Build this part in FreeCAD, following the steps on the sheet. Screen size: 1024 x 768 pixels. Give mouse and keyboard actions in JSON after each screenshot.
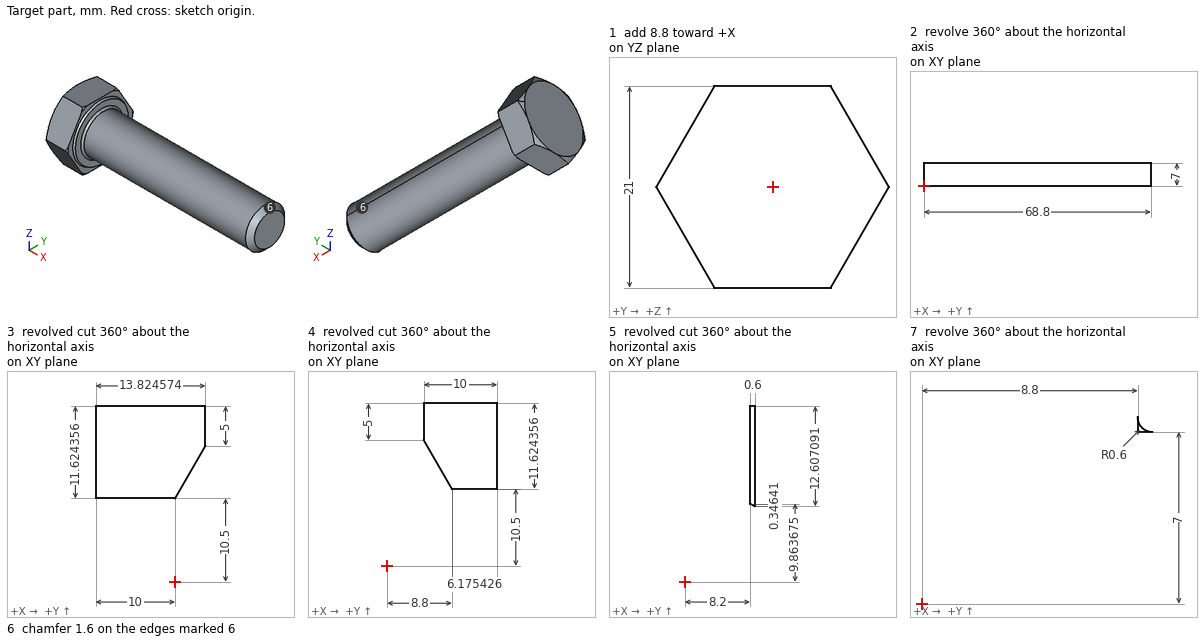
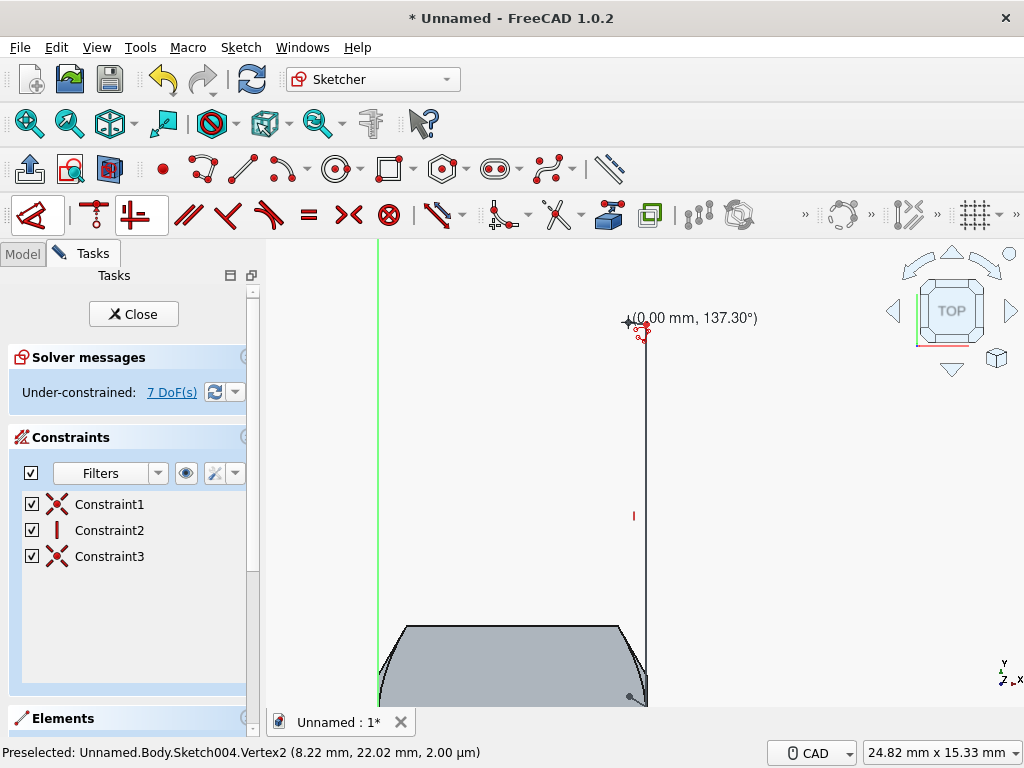
{"action": "scroll", "coordinate": [629, 322], "scroll_direction": "down", "scroll_amount": 4}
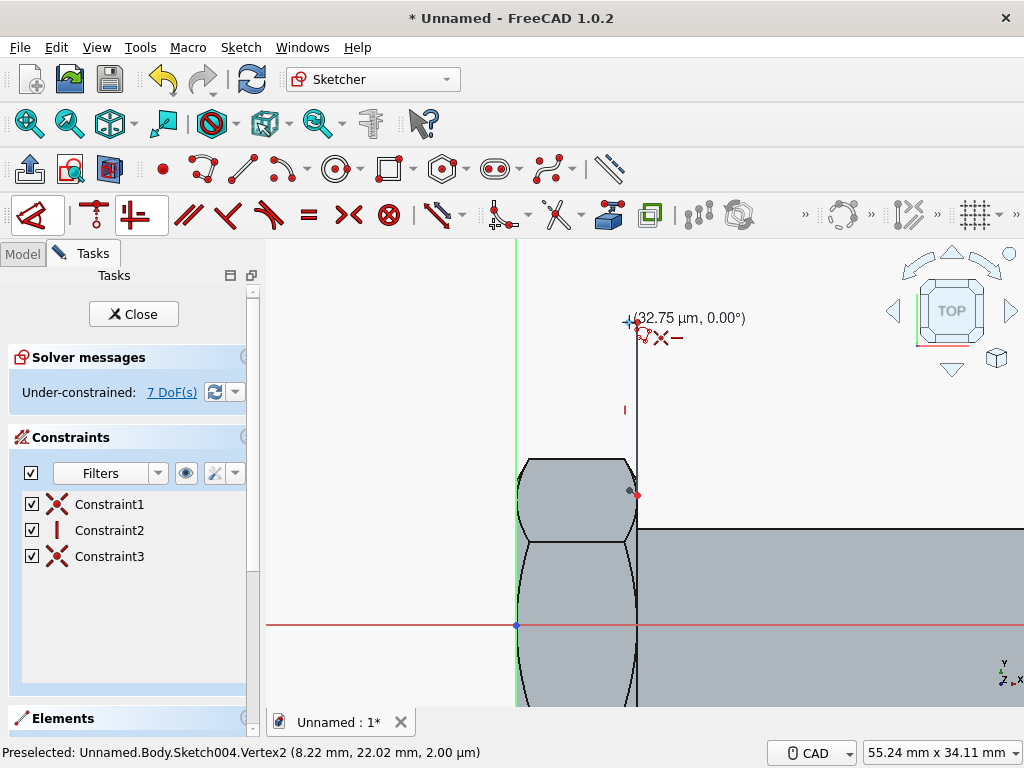
{"action": "scroll", "coordinate": [629, 490], "scroll_direction": "up", "scroll_amount": 7}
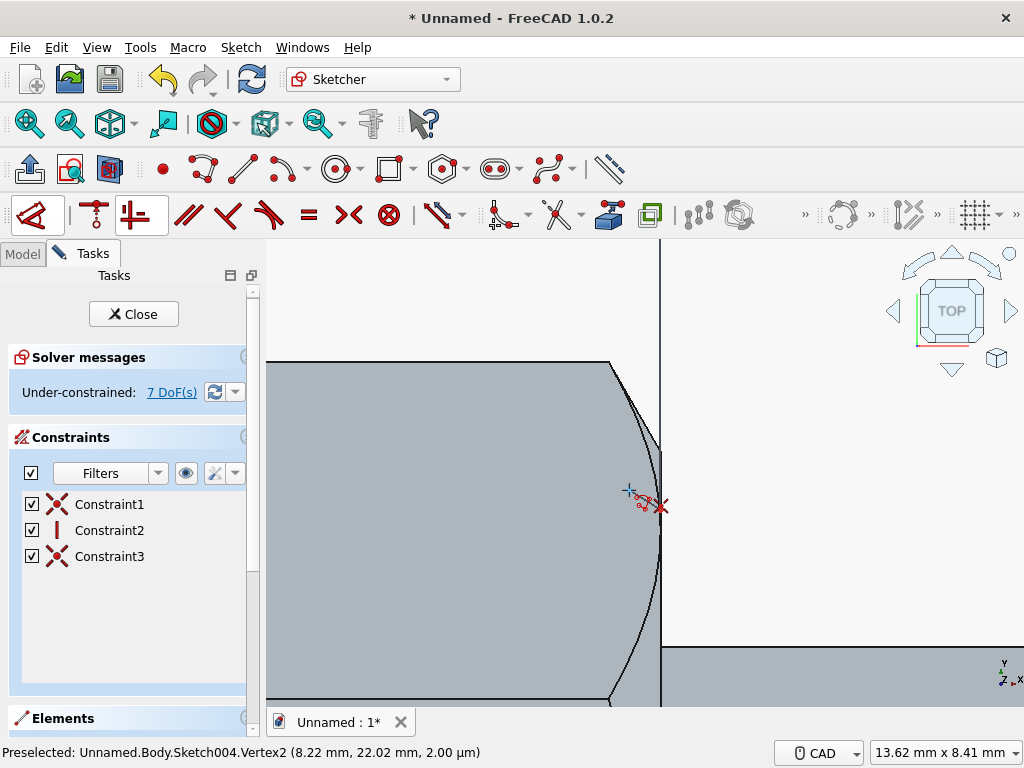
{"action": "left_click", "coordinate": [629, 490]}
{"action": "key", "text": "Escape"}
{"action": "key", "text": "Escape"}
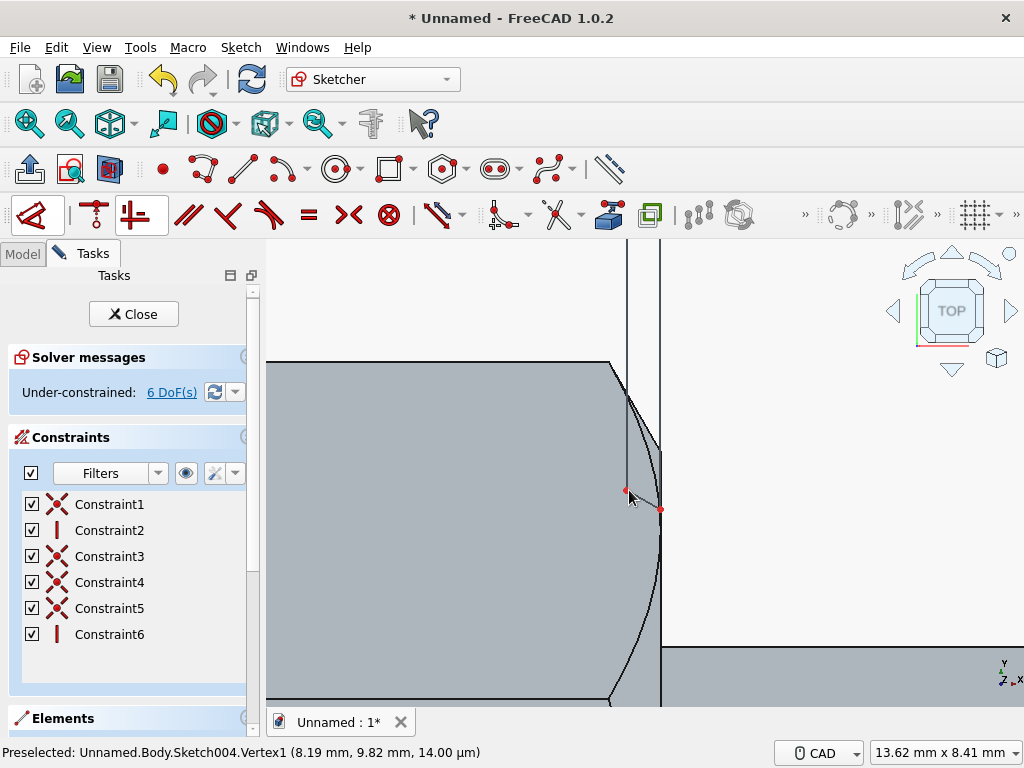
{"action": "scroll", "coordinate": [629, 490], "scroll_direction": "down", "scroll_amount": 7}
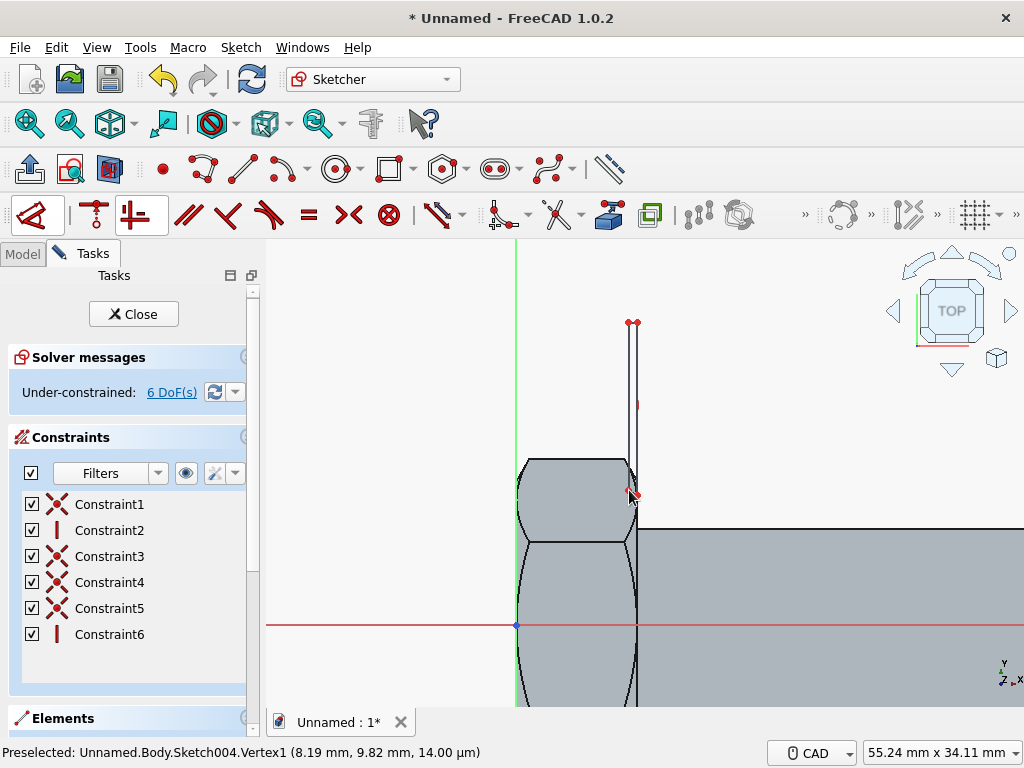
{"action": "scroll", "coordinate": [635, 323], "scroll_direction": "up", "scroll_amount": 9}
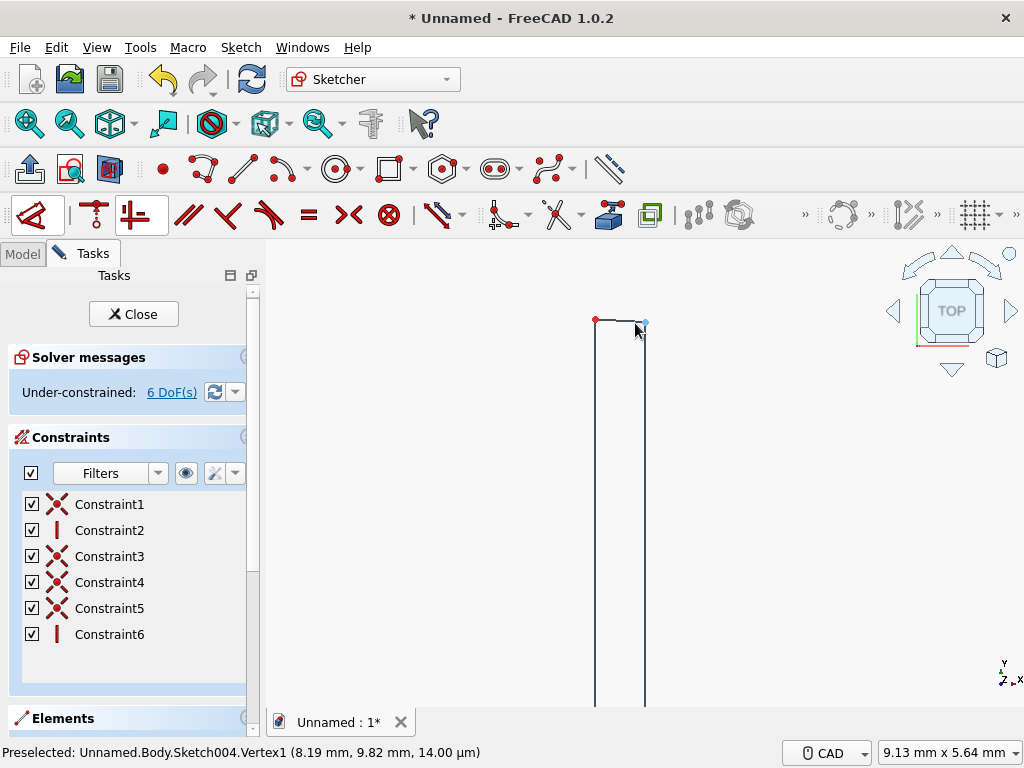
{"action": "left_click", "coordinate": [630, 321]}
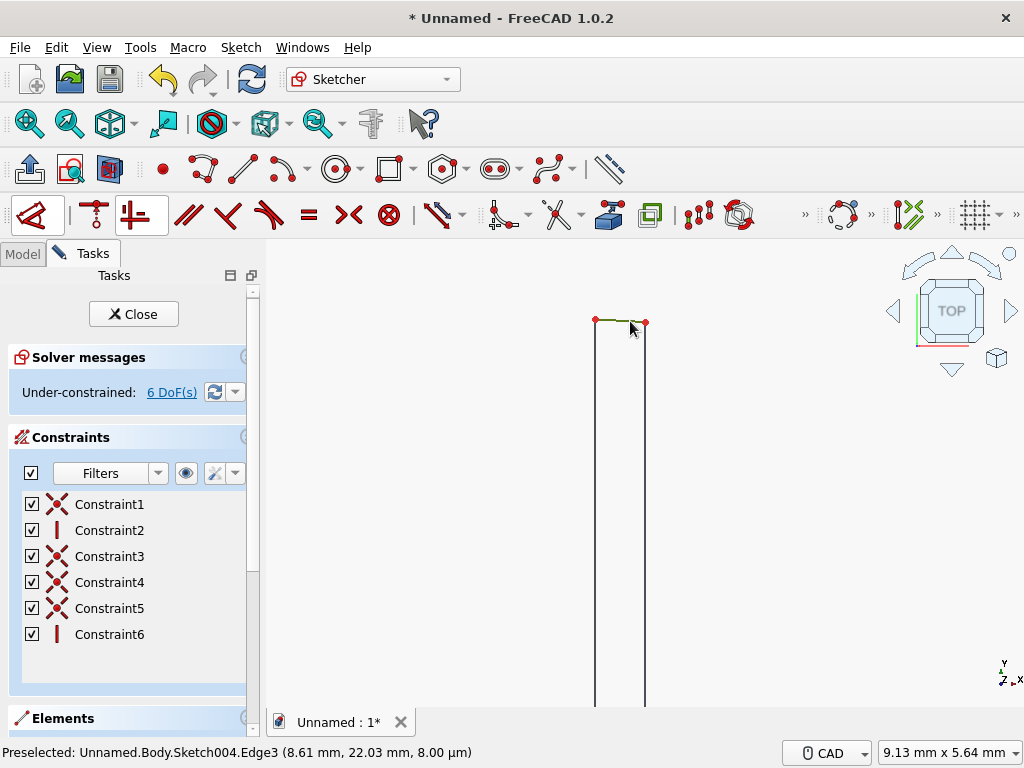
{"action": "key", "text": "h"}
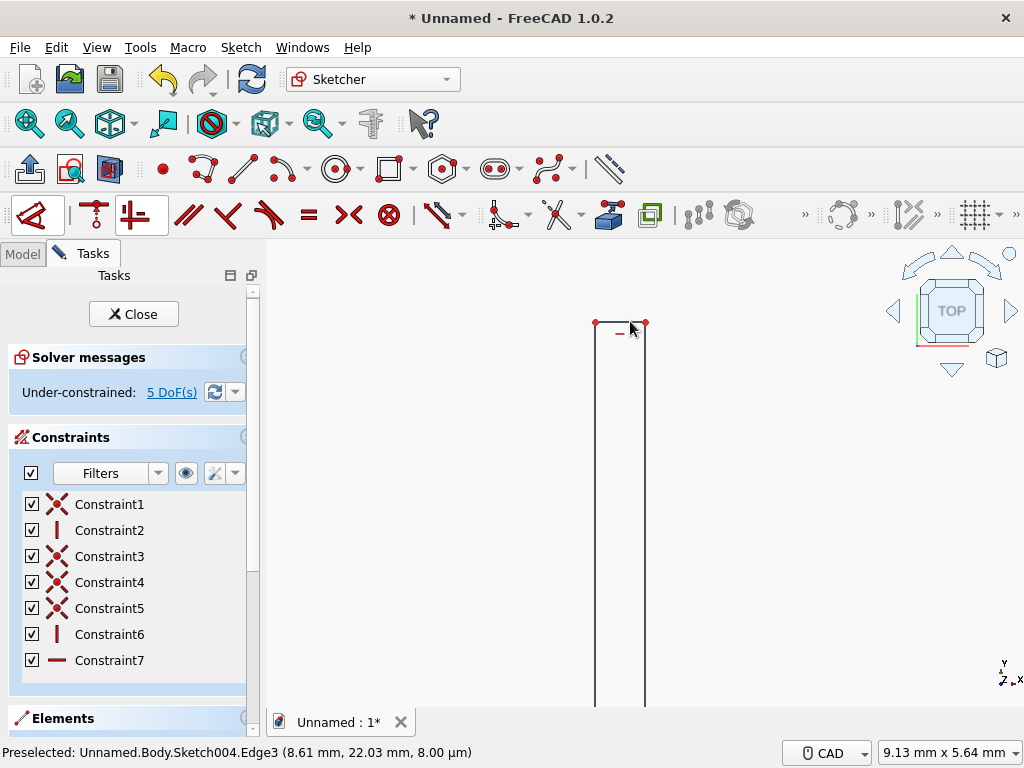
{"action": "left_click", "coordinate": [630, 322]}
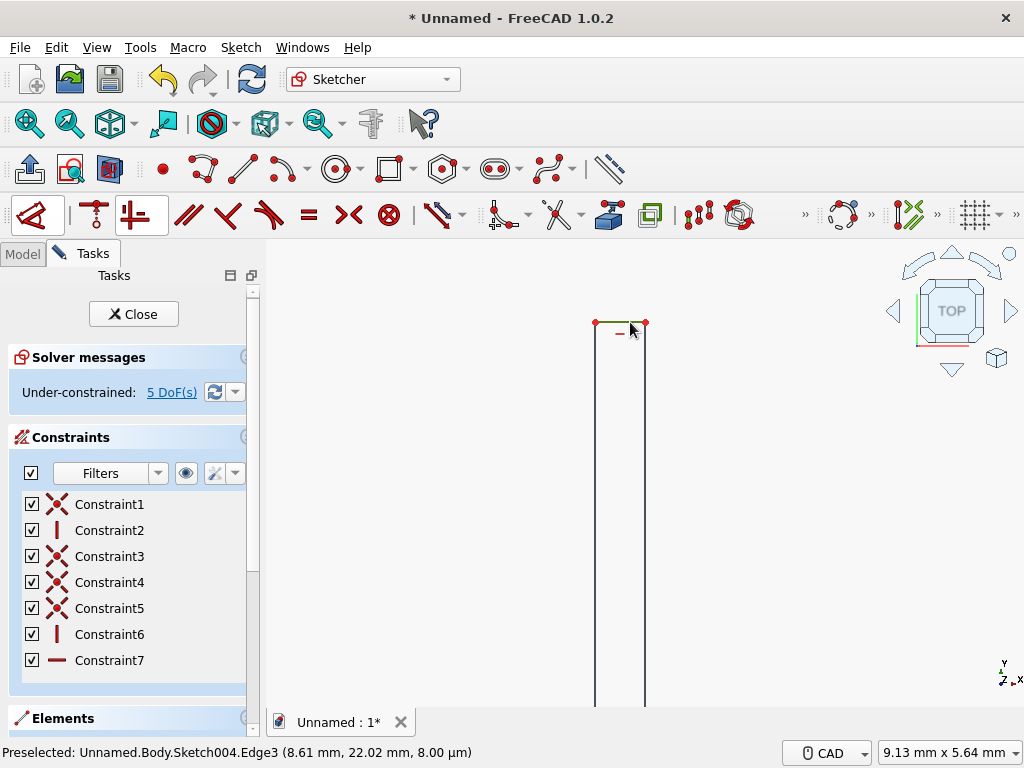
{"action": "left_click", "coordinate": [58, 216]}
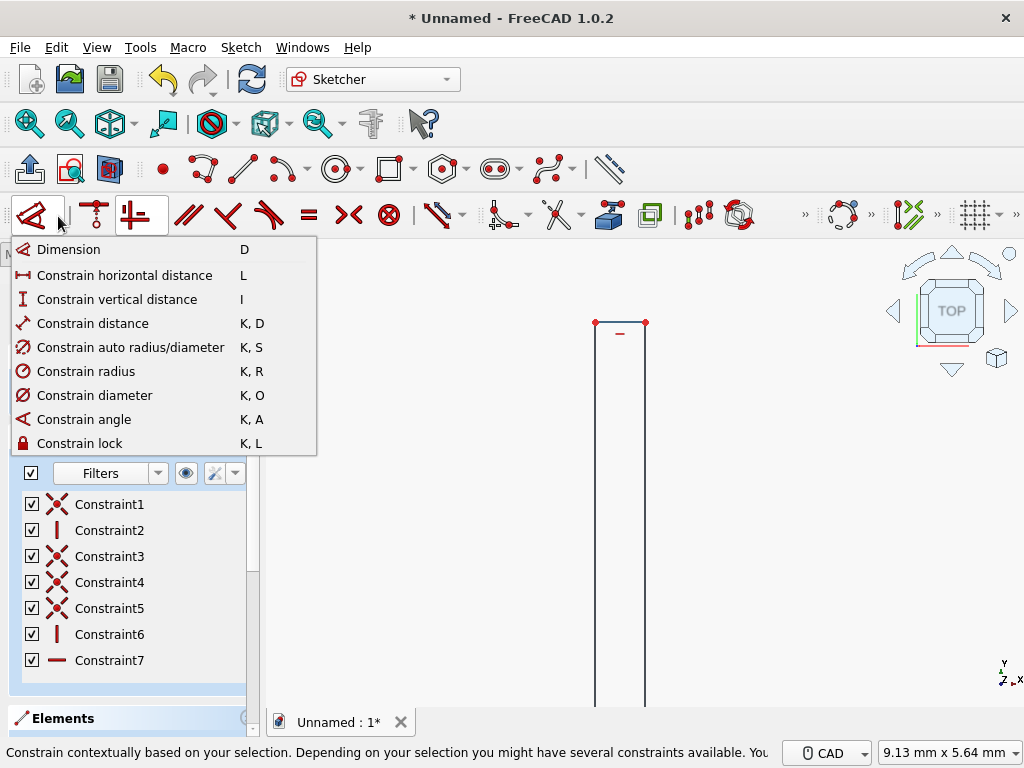
{"action": "left_click", "coordinate": [164, 275]}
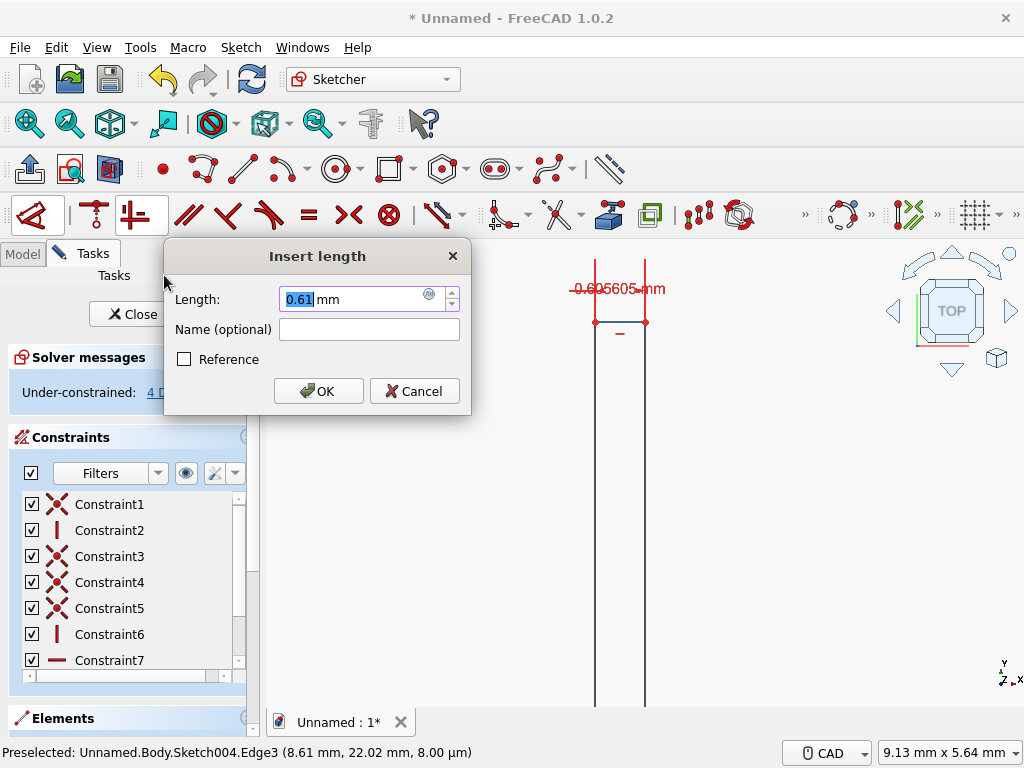
{"action": "type", "text": "0.6"}
{"action": "key", "text": "Return"}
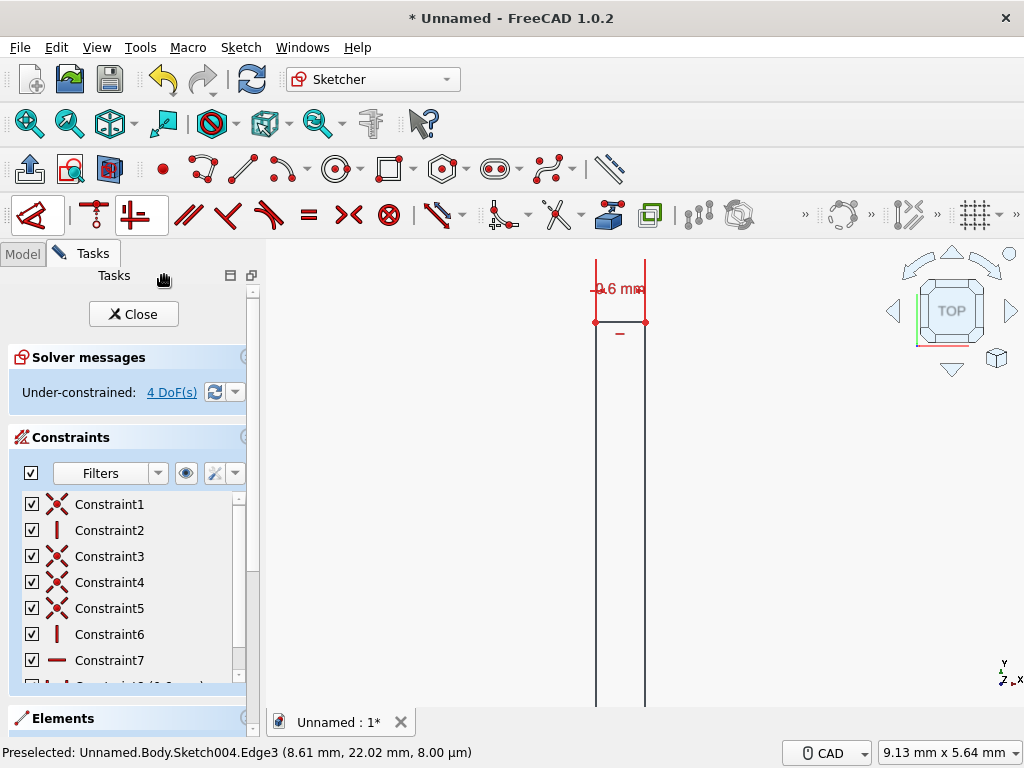
{"action": "scroll", "coordinate": [635, 323], "scroll_direction": "down", "scroll_amount": 9}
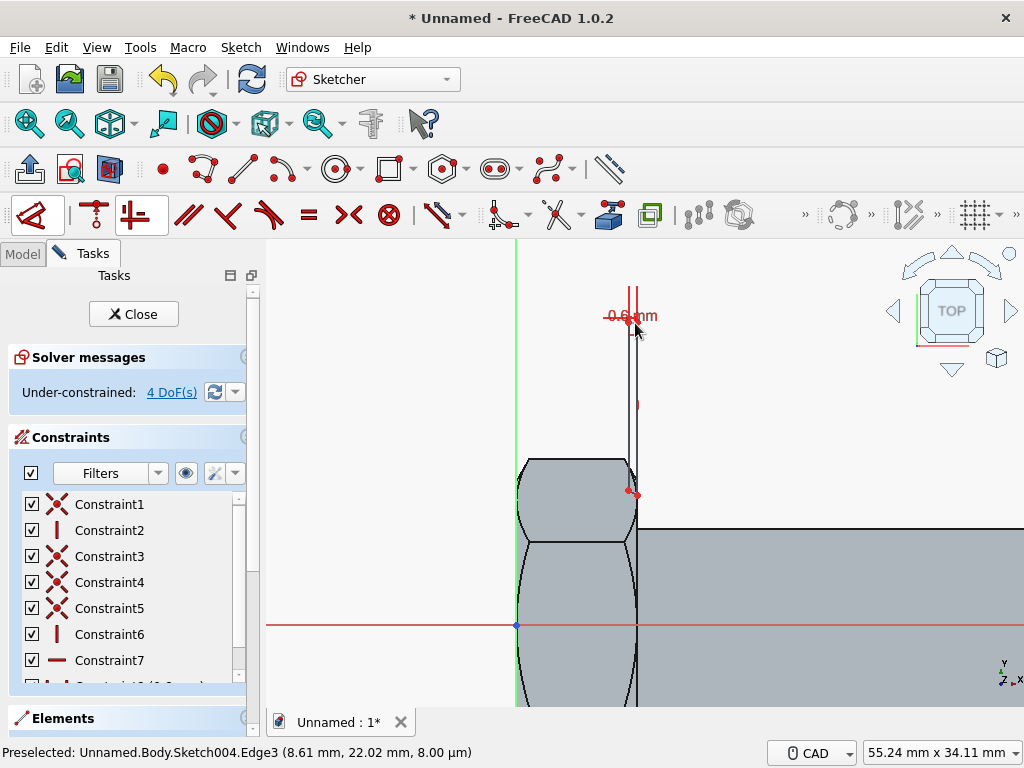
{"action": "scroll", "coordinate": [629, 490], "scroll_direction": "up", "scroll_amount": 2}